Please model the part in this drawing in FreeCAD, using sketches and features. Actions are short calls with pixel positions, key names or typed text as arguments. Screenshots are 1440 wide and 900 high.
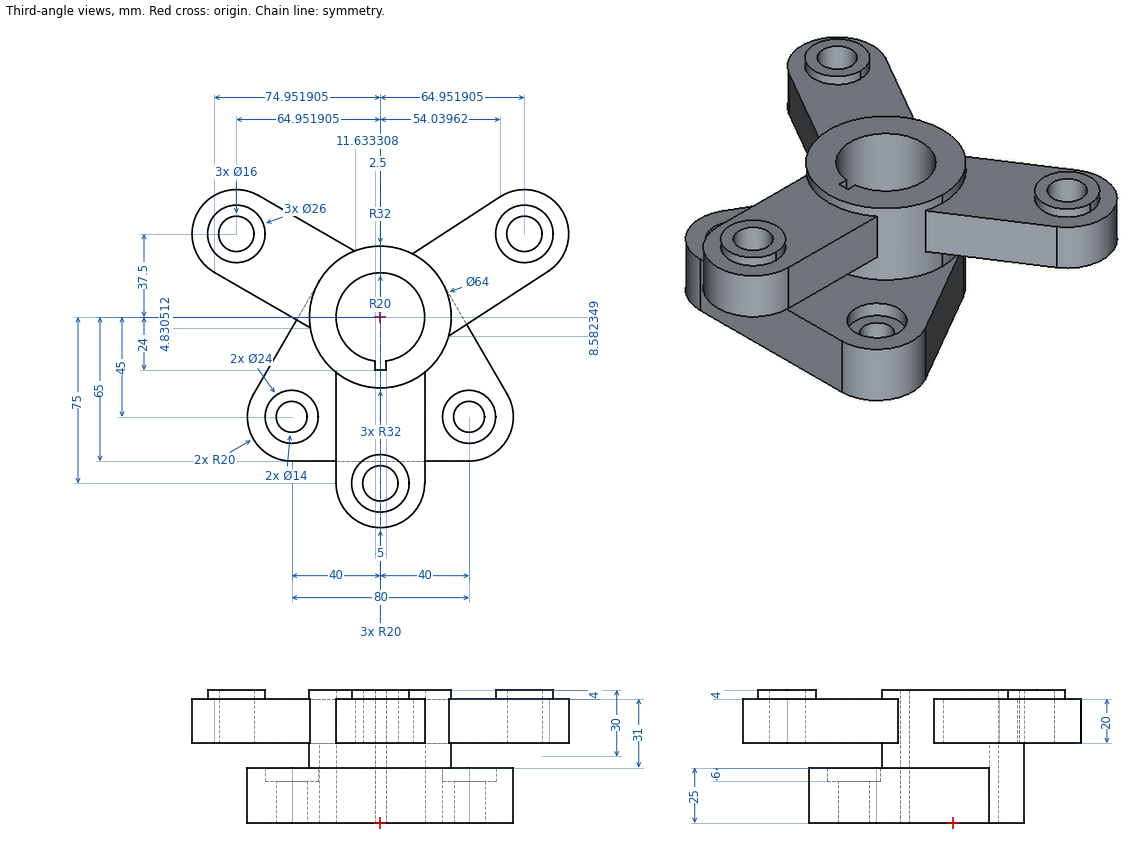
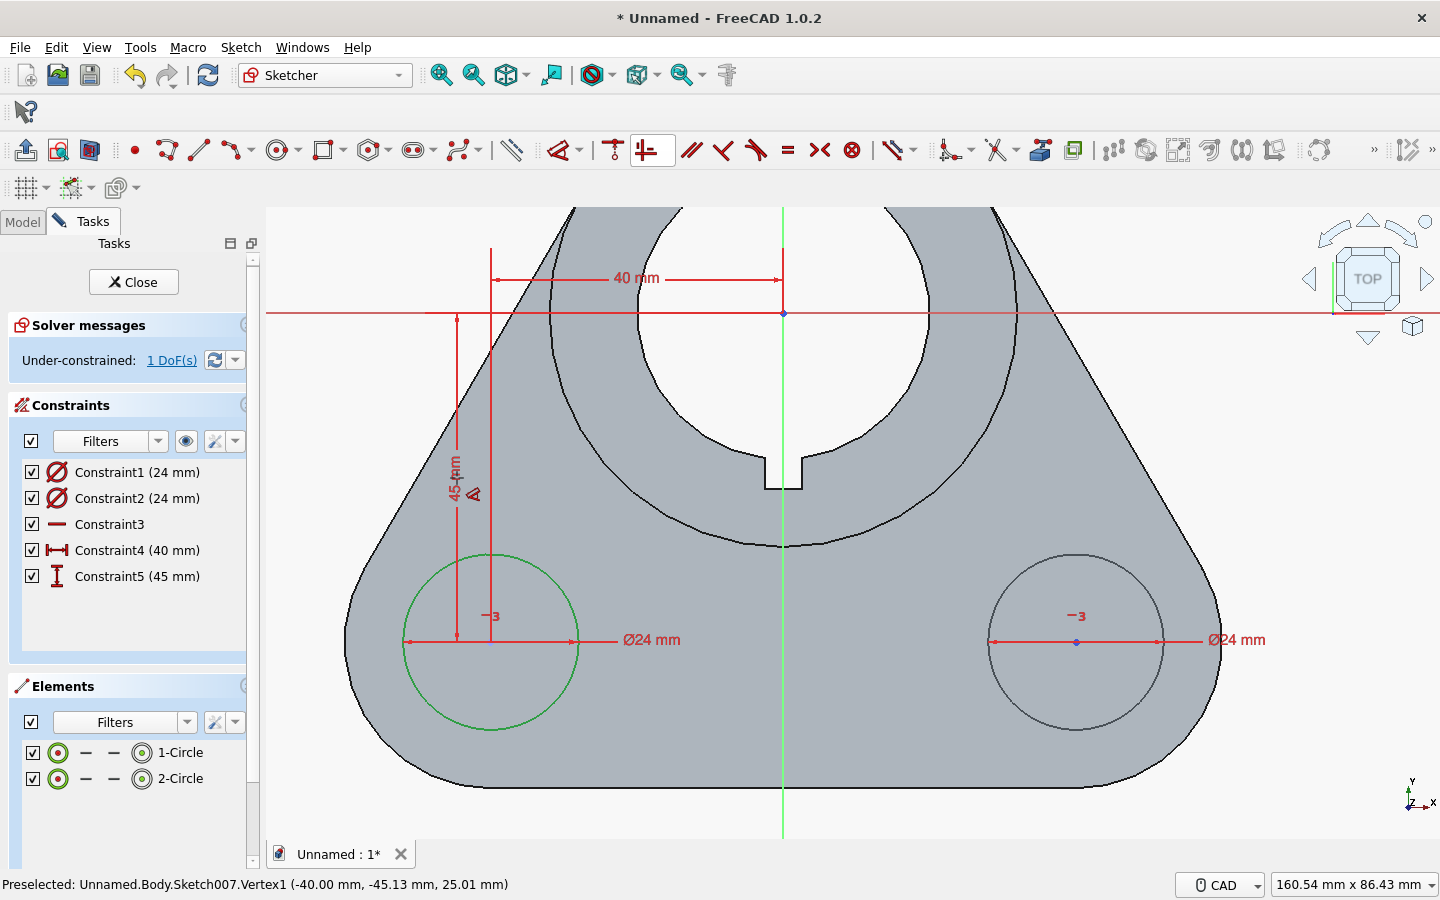
click(1076, 642)
click(930, 279)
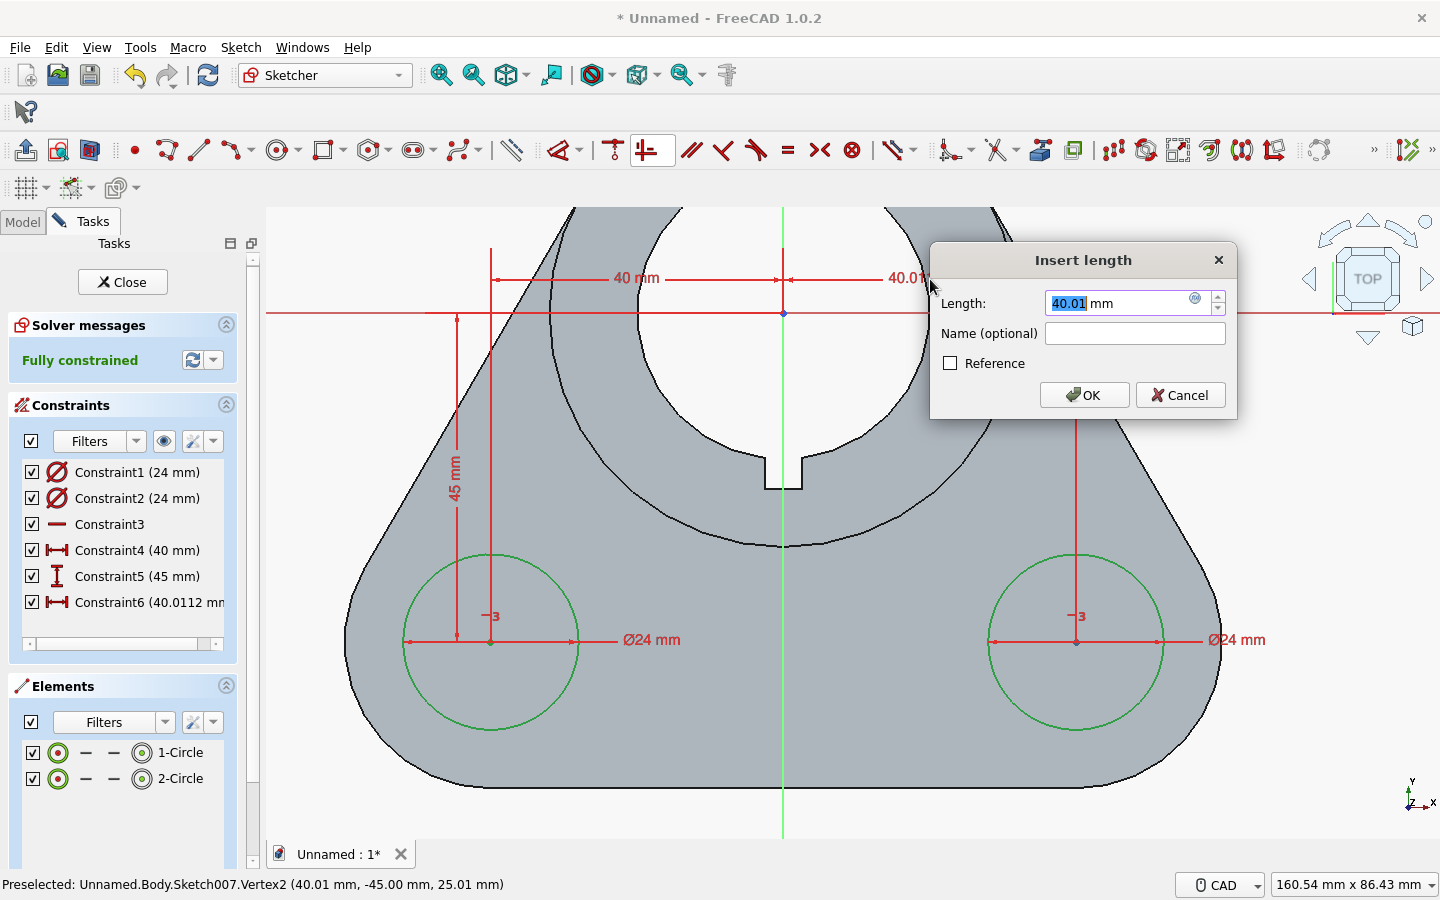
text(40)
key(Return)
key(Escape)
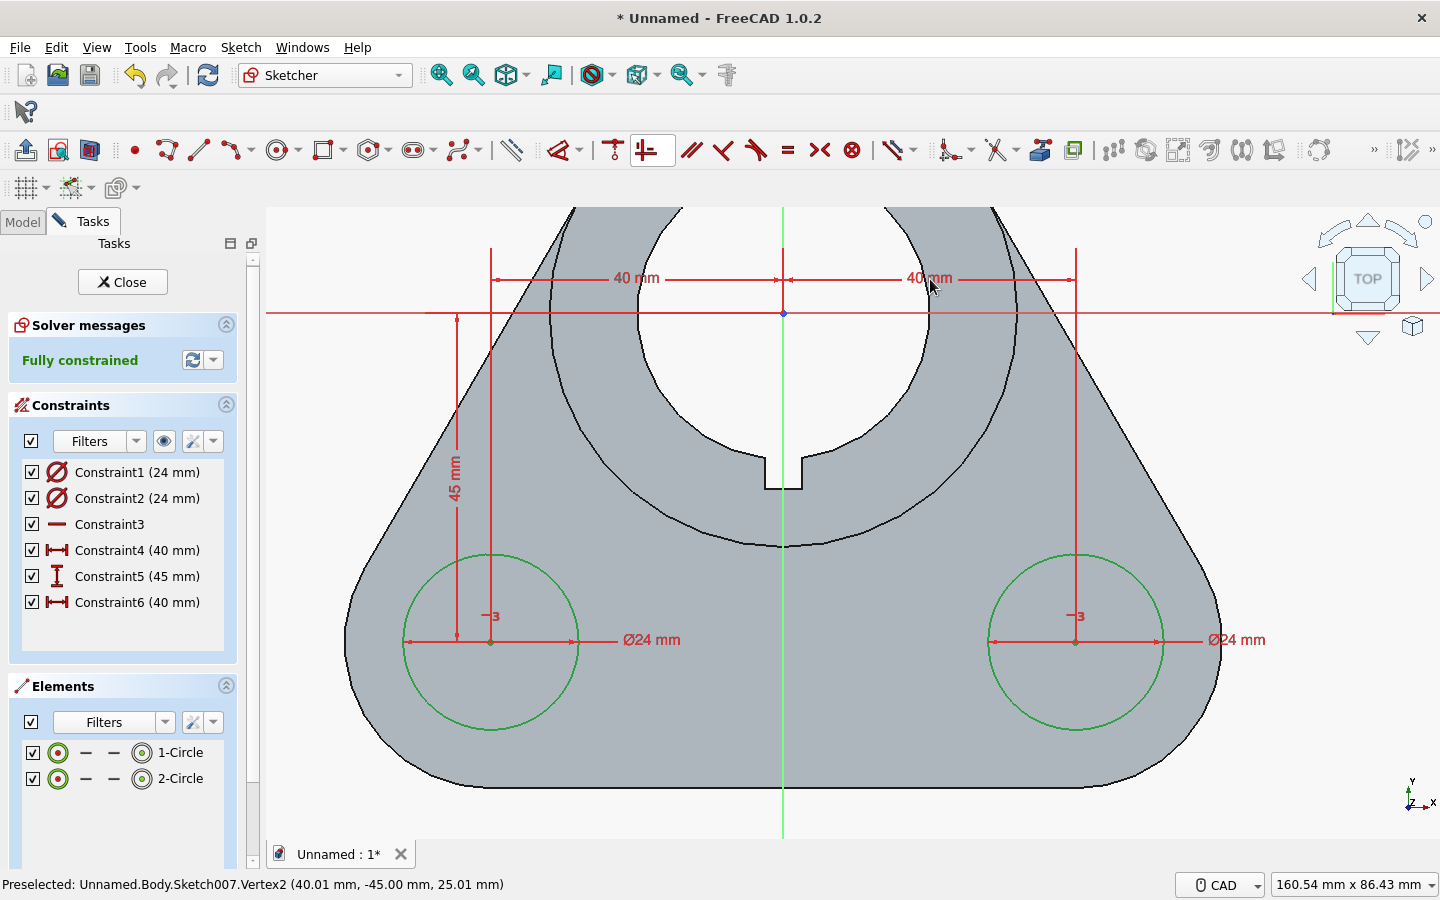
click(123, 282)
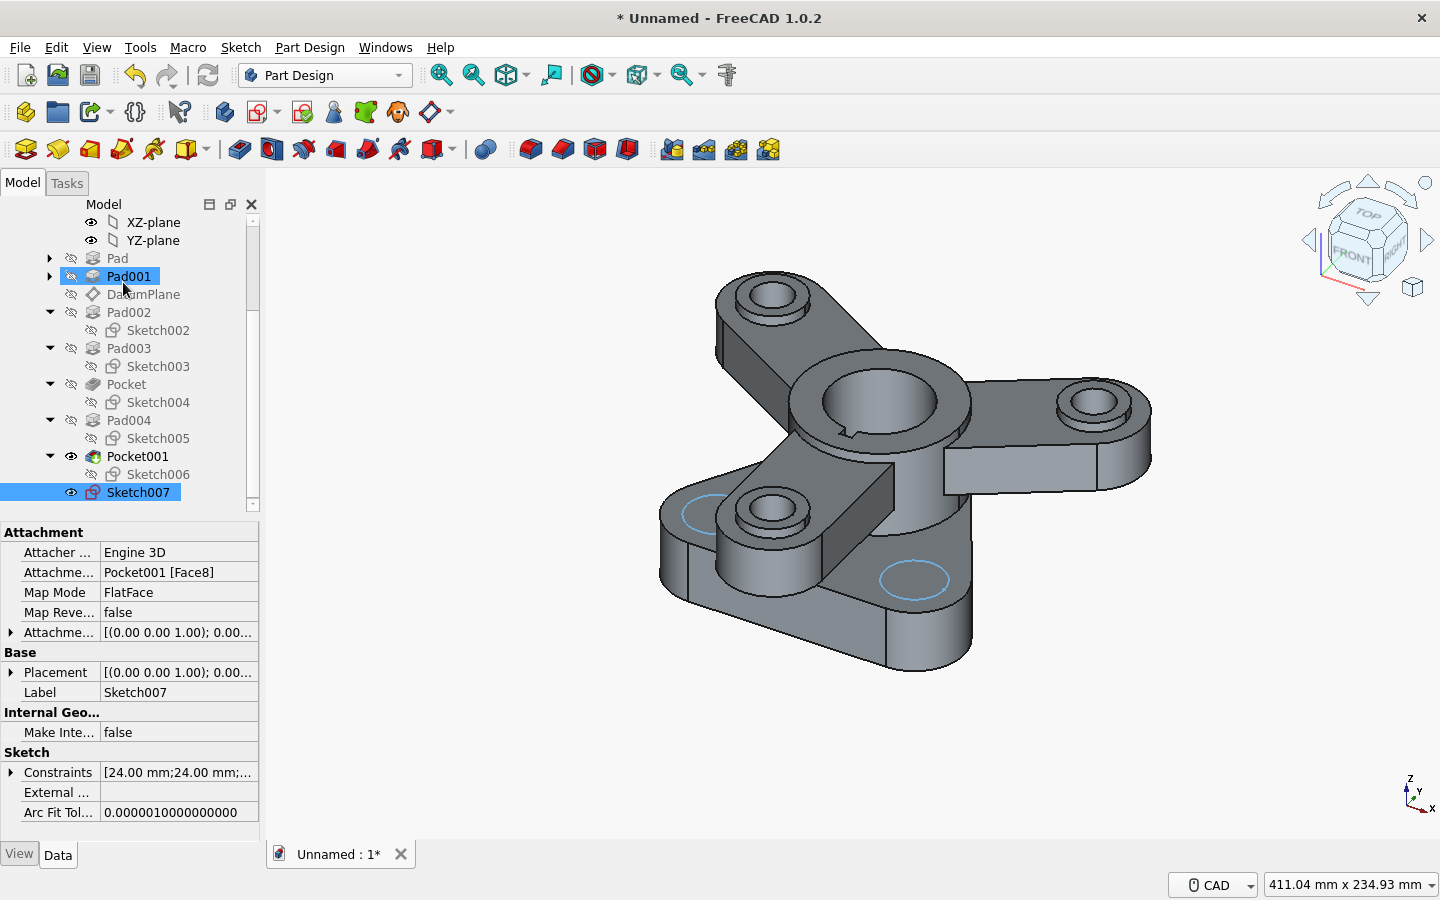
click(240, 150)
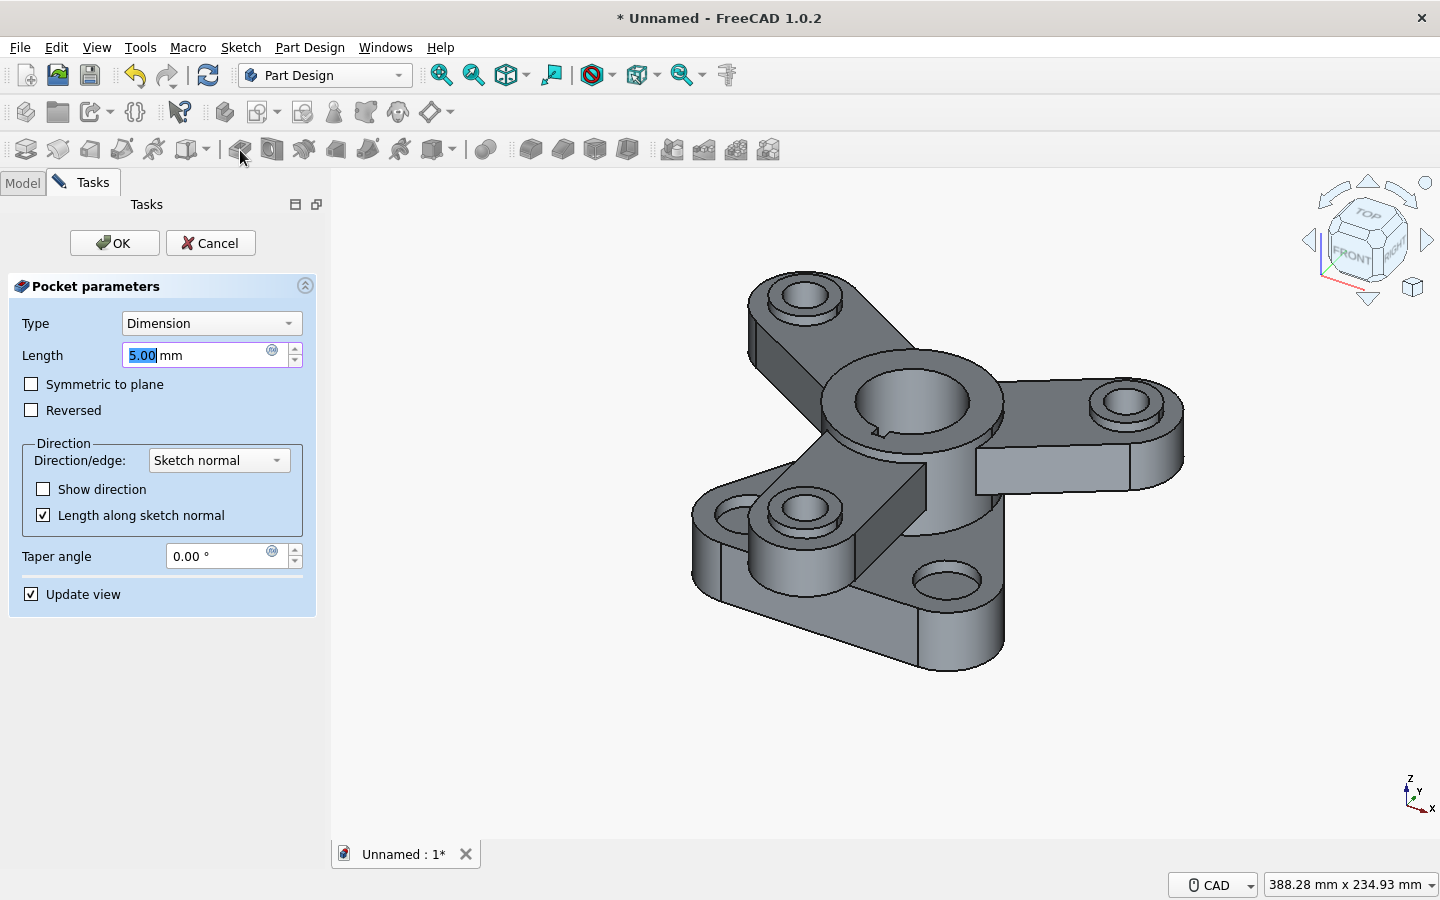
text(6)
key(Tab)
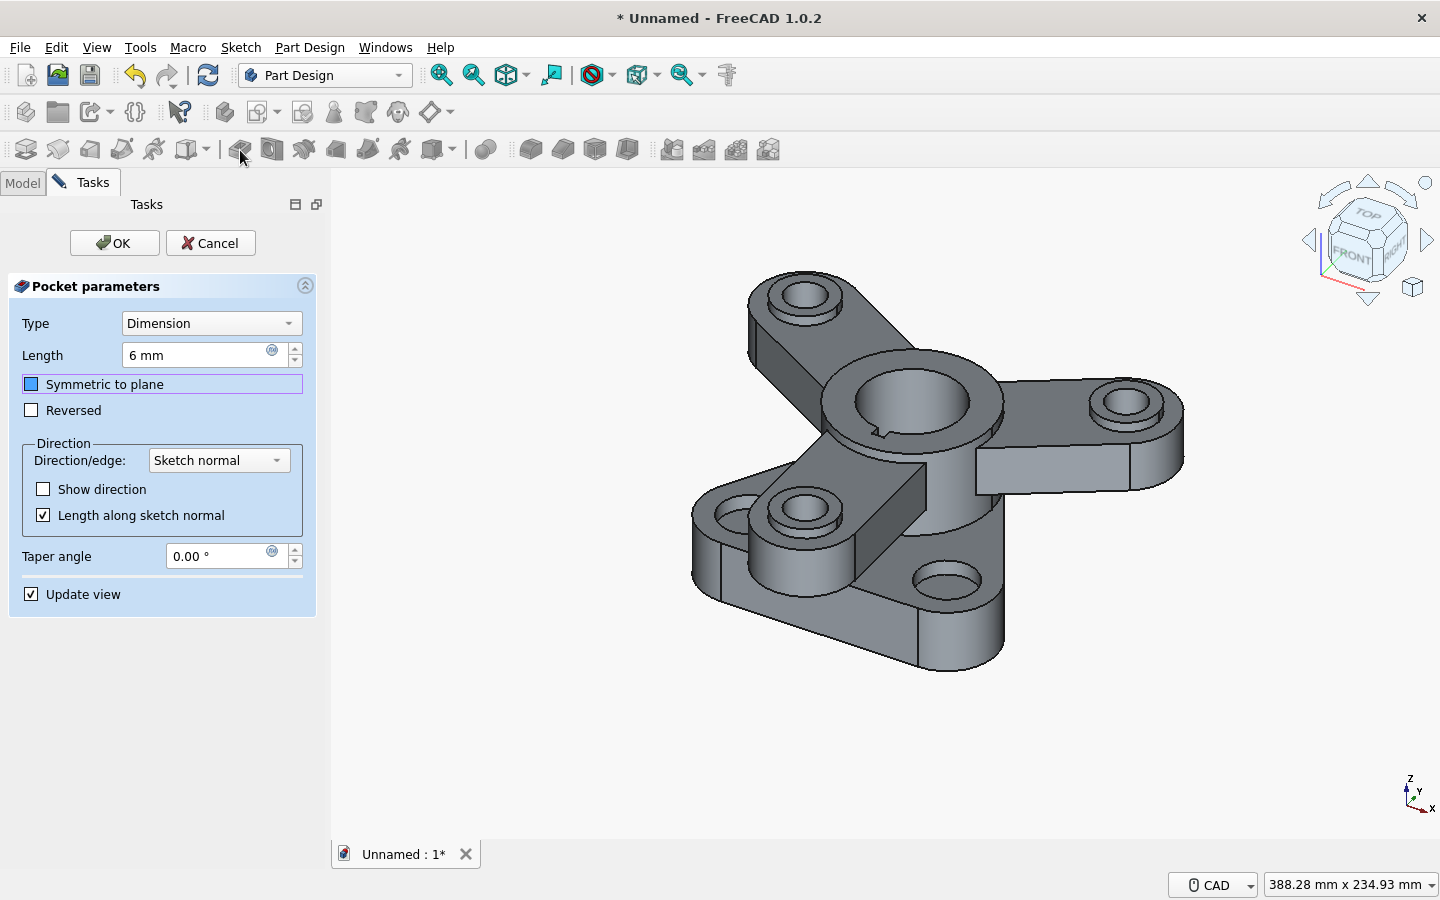
click(115, 243)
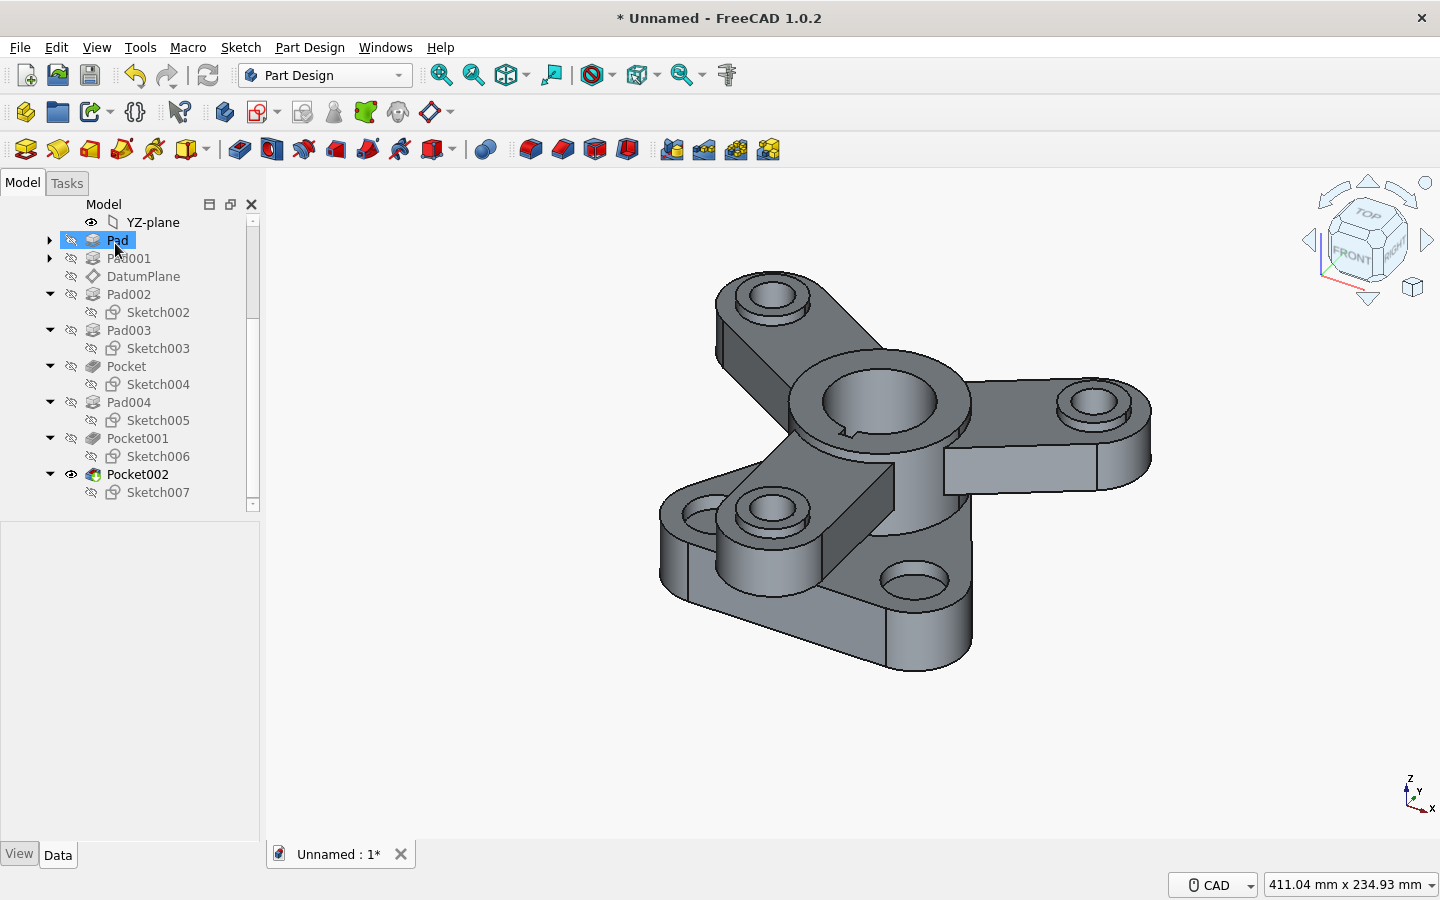
click(919, 588)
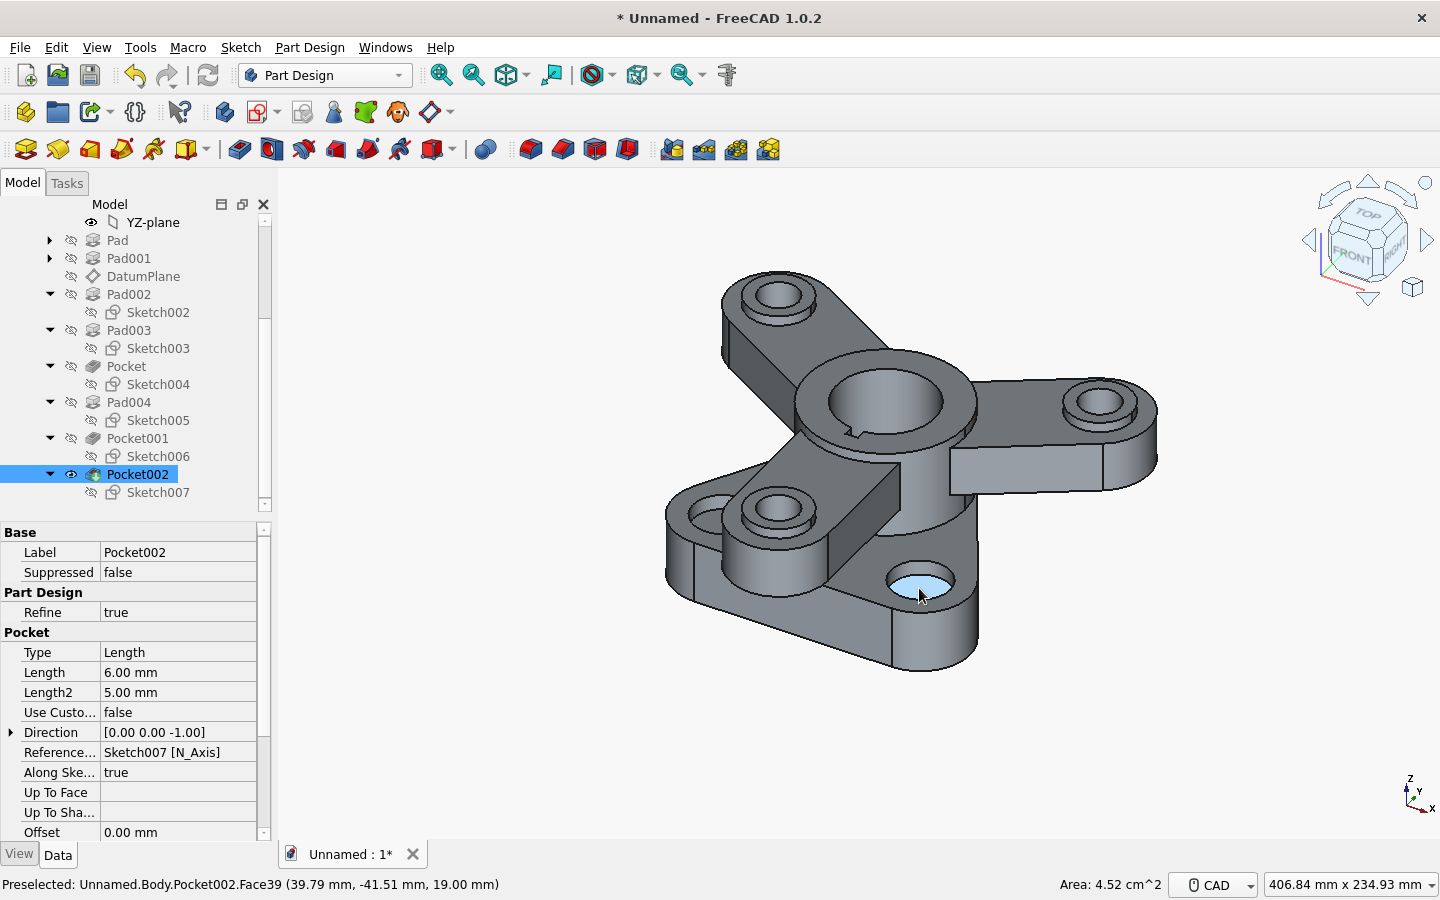
click(258, 112)